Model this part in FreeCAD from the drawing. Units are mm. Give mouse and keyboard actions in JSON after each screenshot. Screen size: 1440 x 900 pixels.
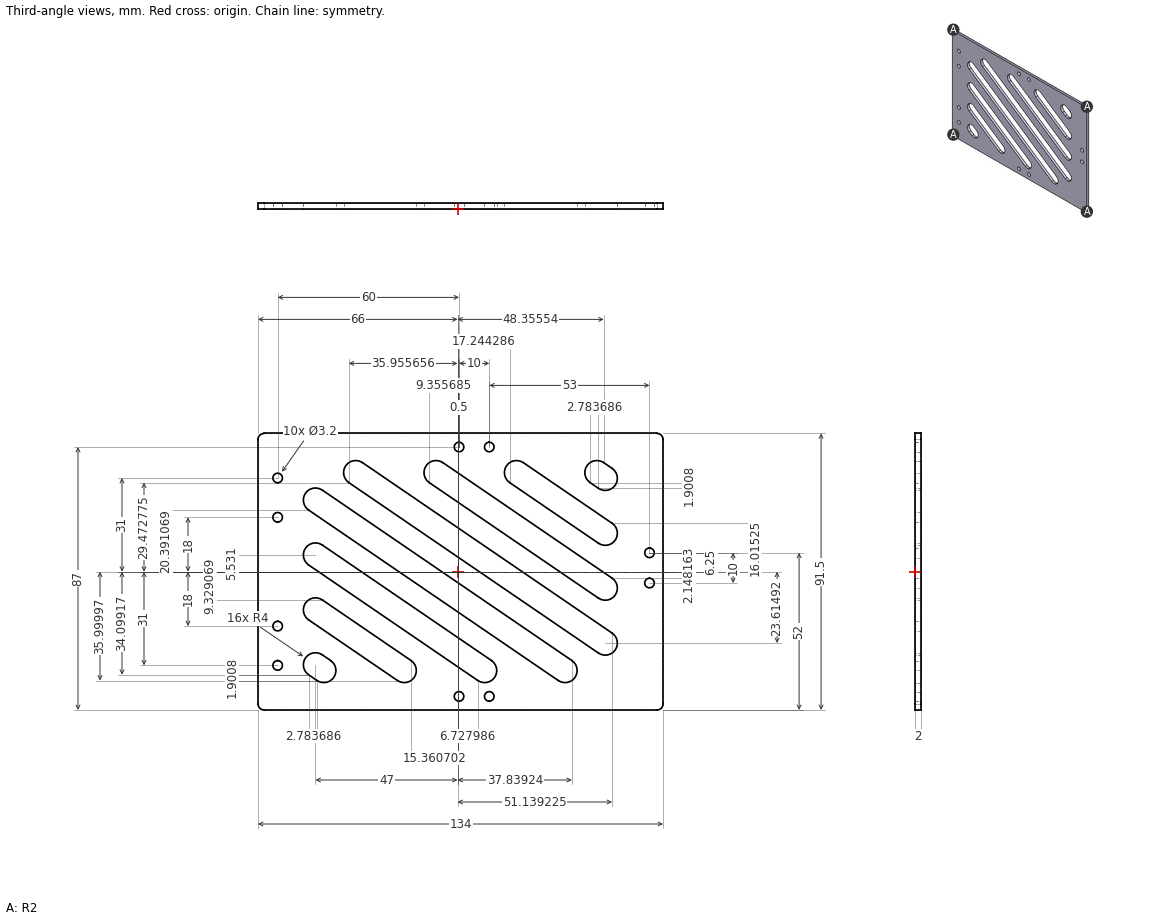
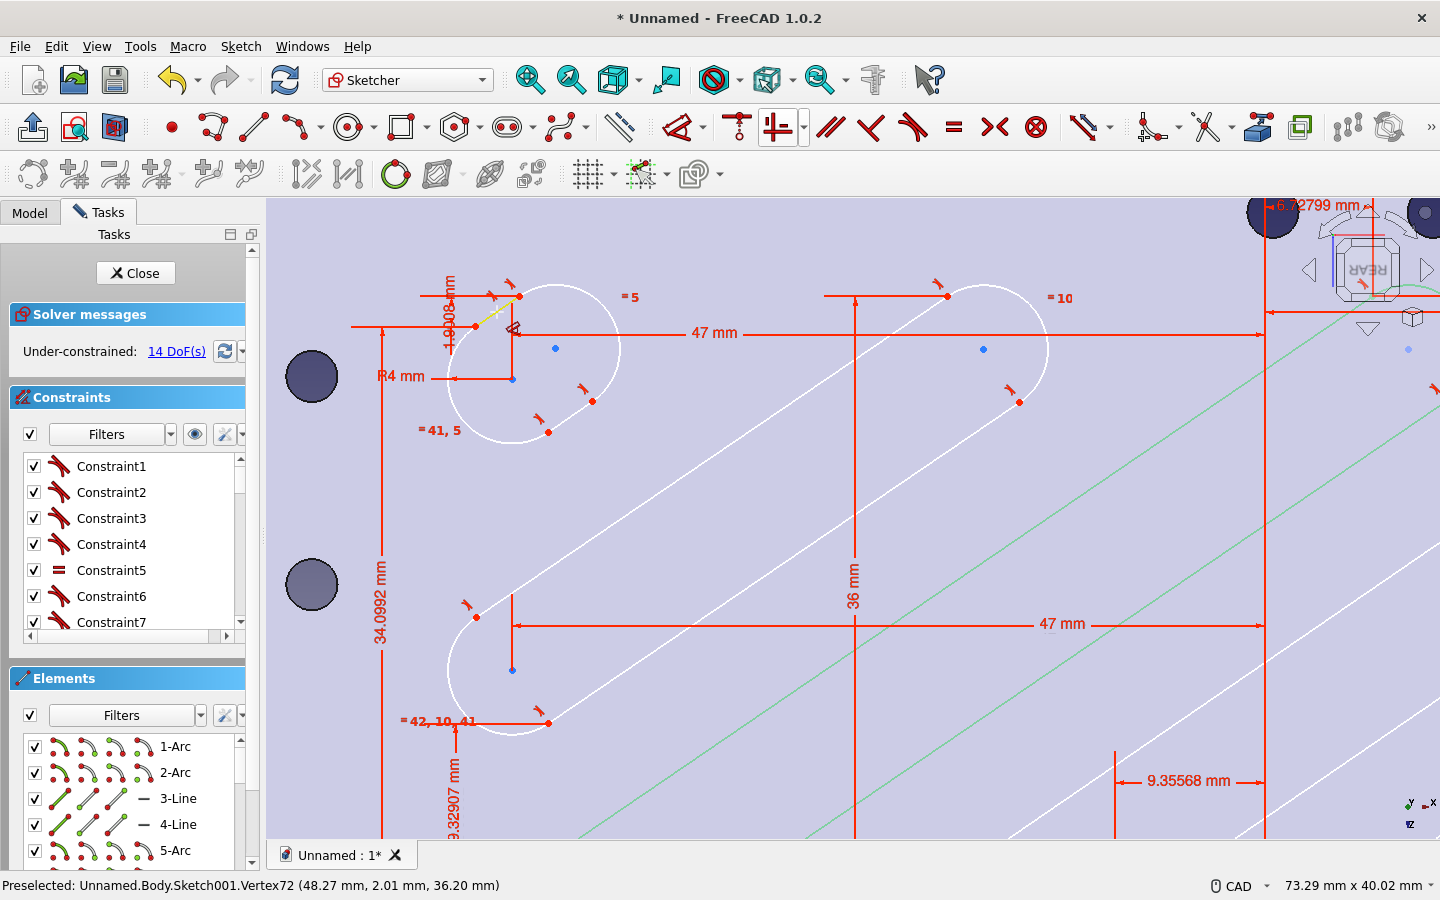
{"action": "left_click", "coordinate": [497, 312]}
{"action": "left_click", "coordinate": [497, 262]}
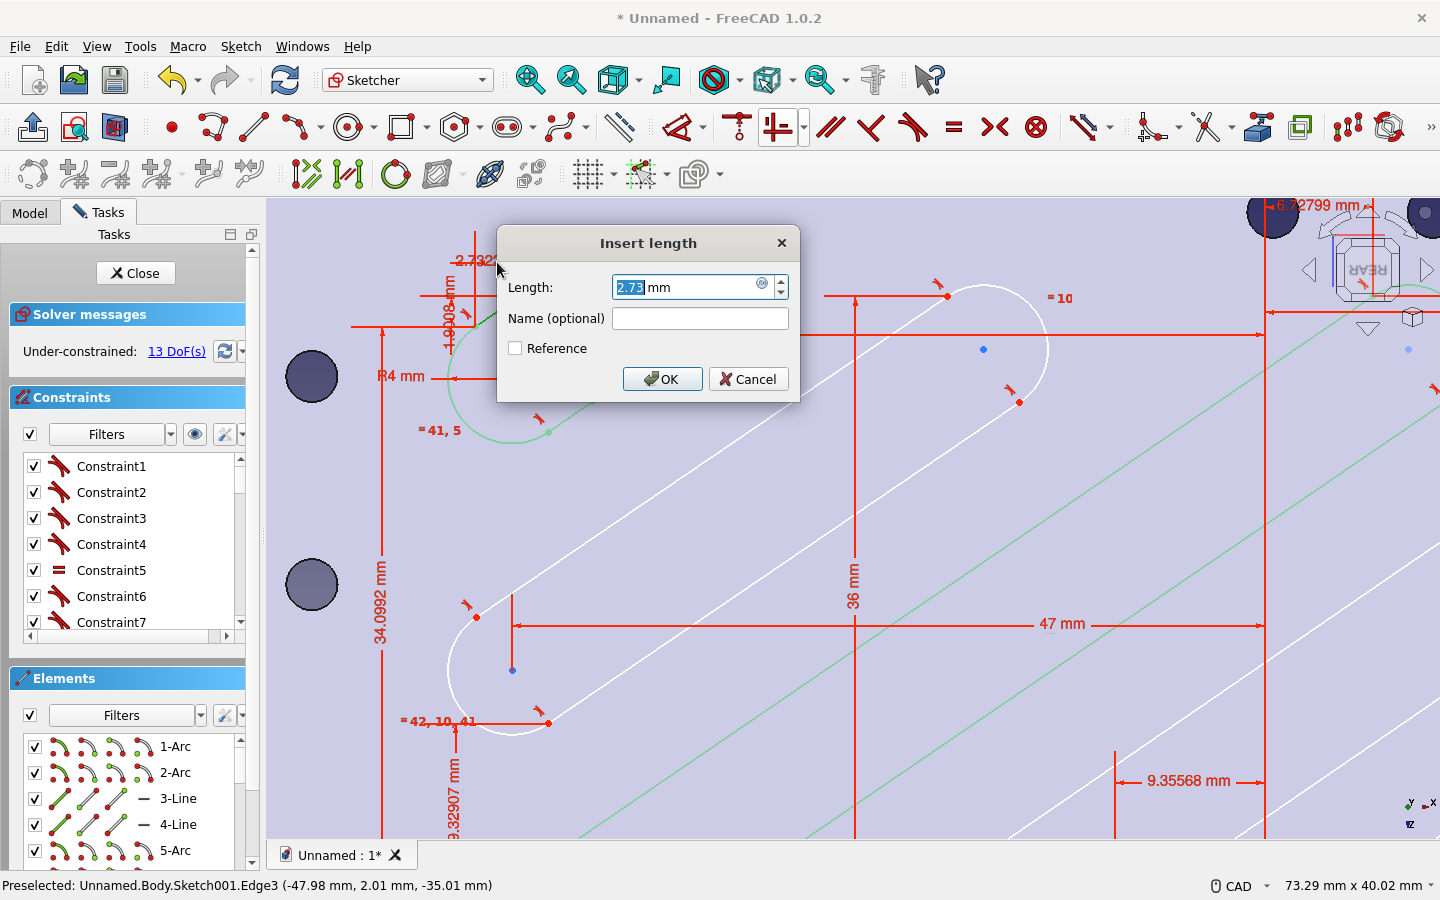
{"action": "type", "text": "2.783686"}
{"action": "key", "text": "Return"}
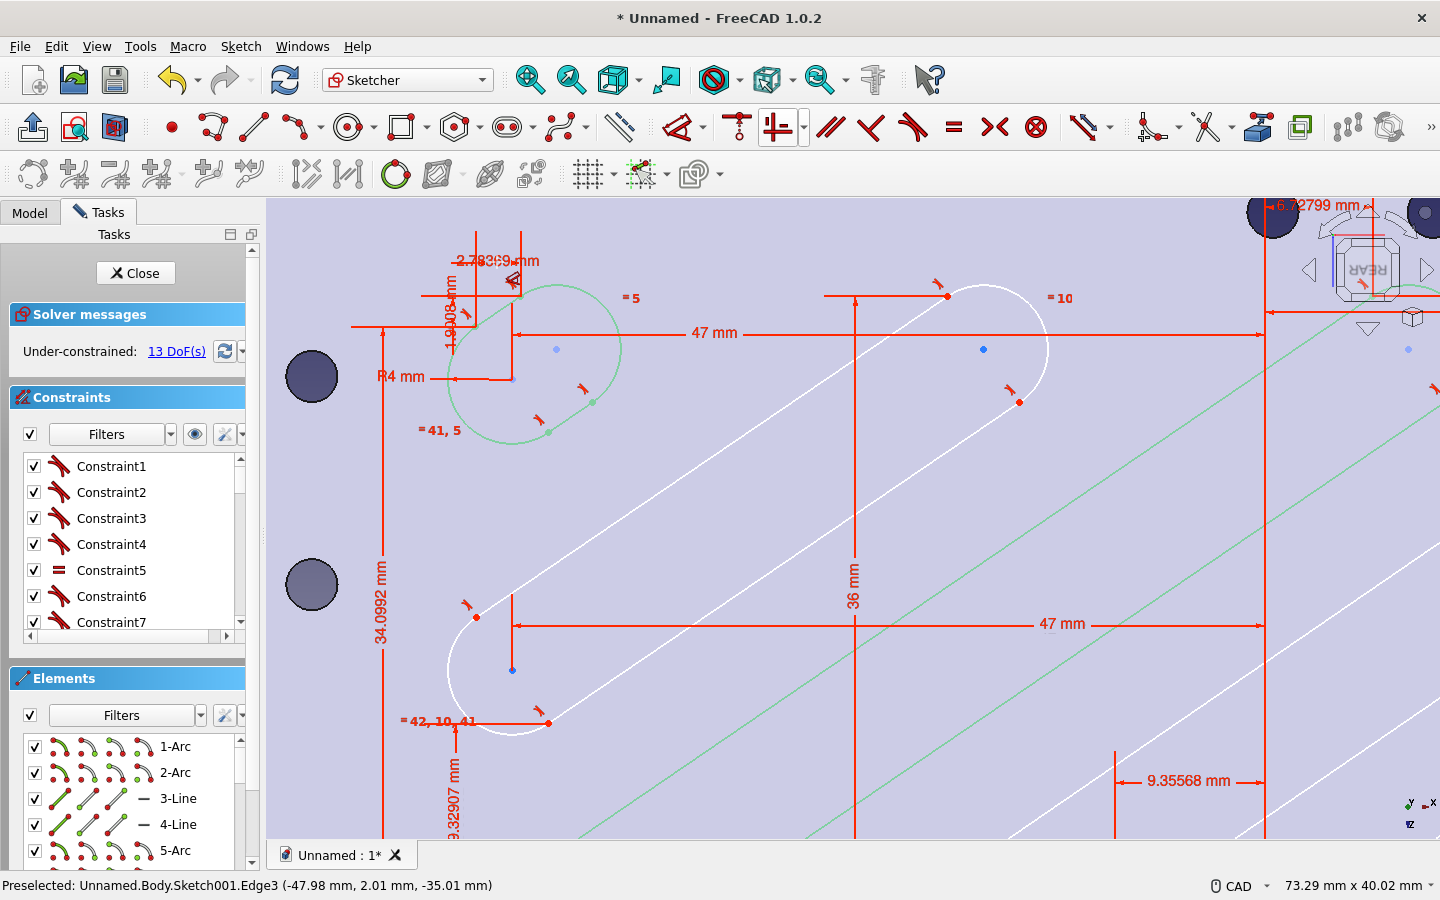
{"action": "scroll", "coordinate": [496, 312], "scroll_direction": "down", "scroll_amount": 5}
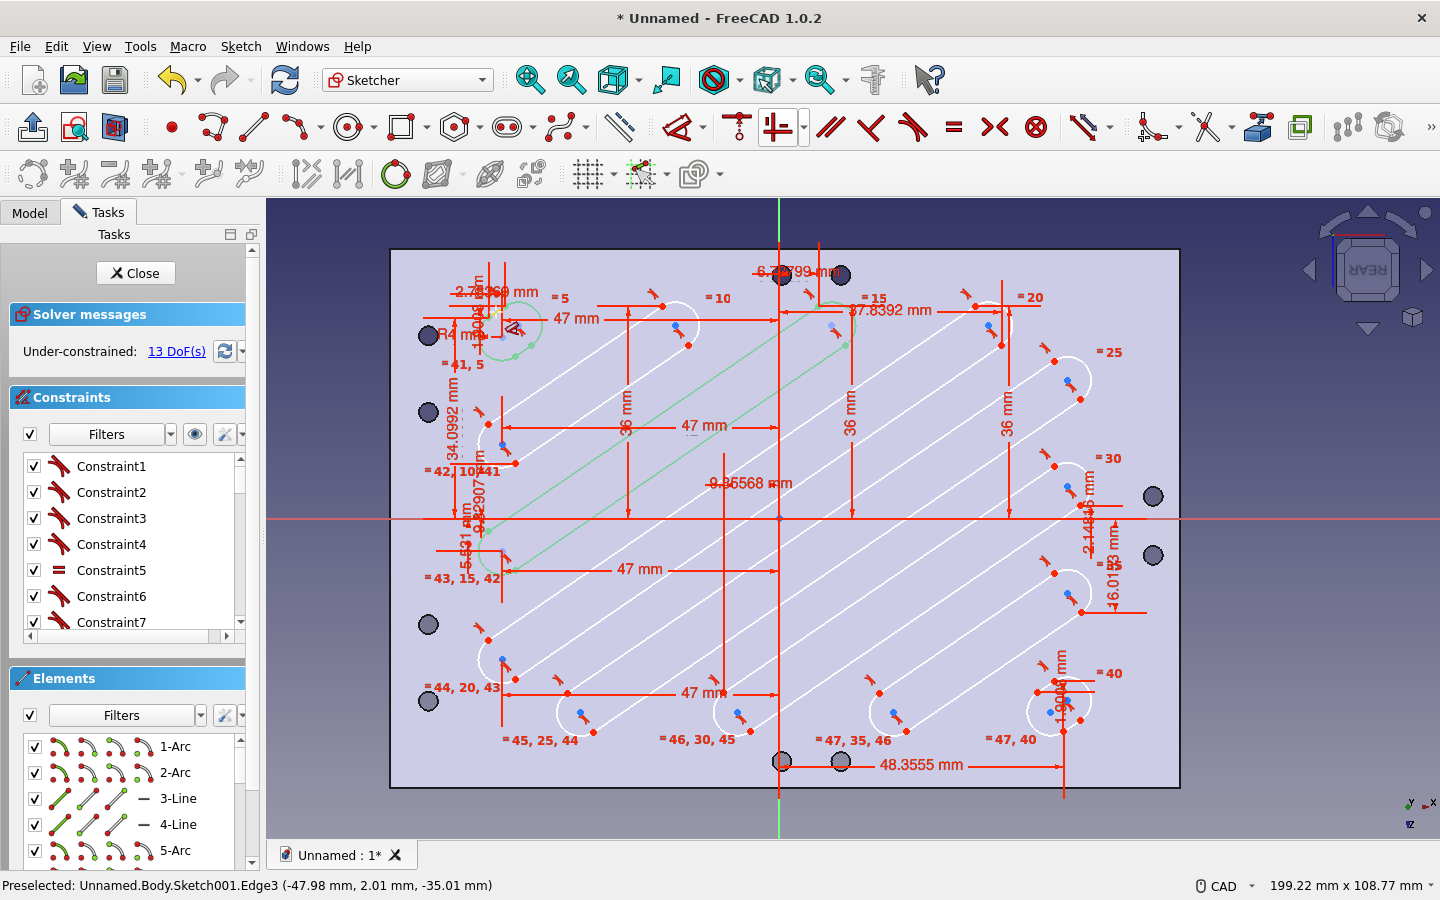
{"action": "scroll", "coordinate": [1043, 689], "scroll_direction": "up", "scroll_amount": 5}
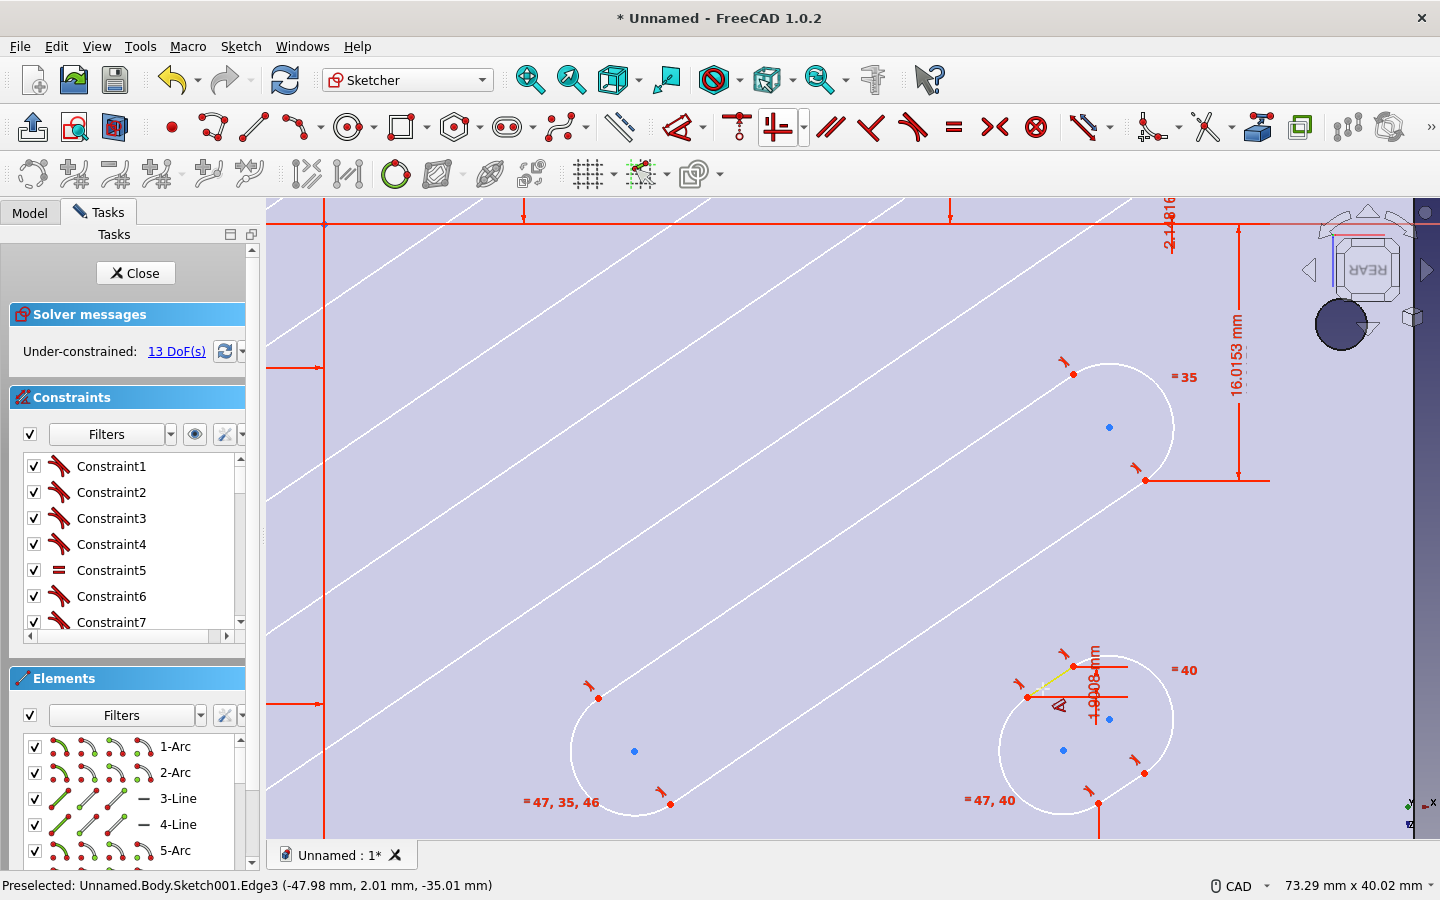
{"action": "left_click", "coordinate": [1042, 688]}
{"action": "left_click", "coordinate": [1051, 731]}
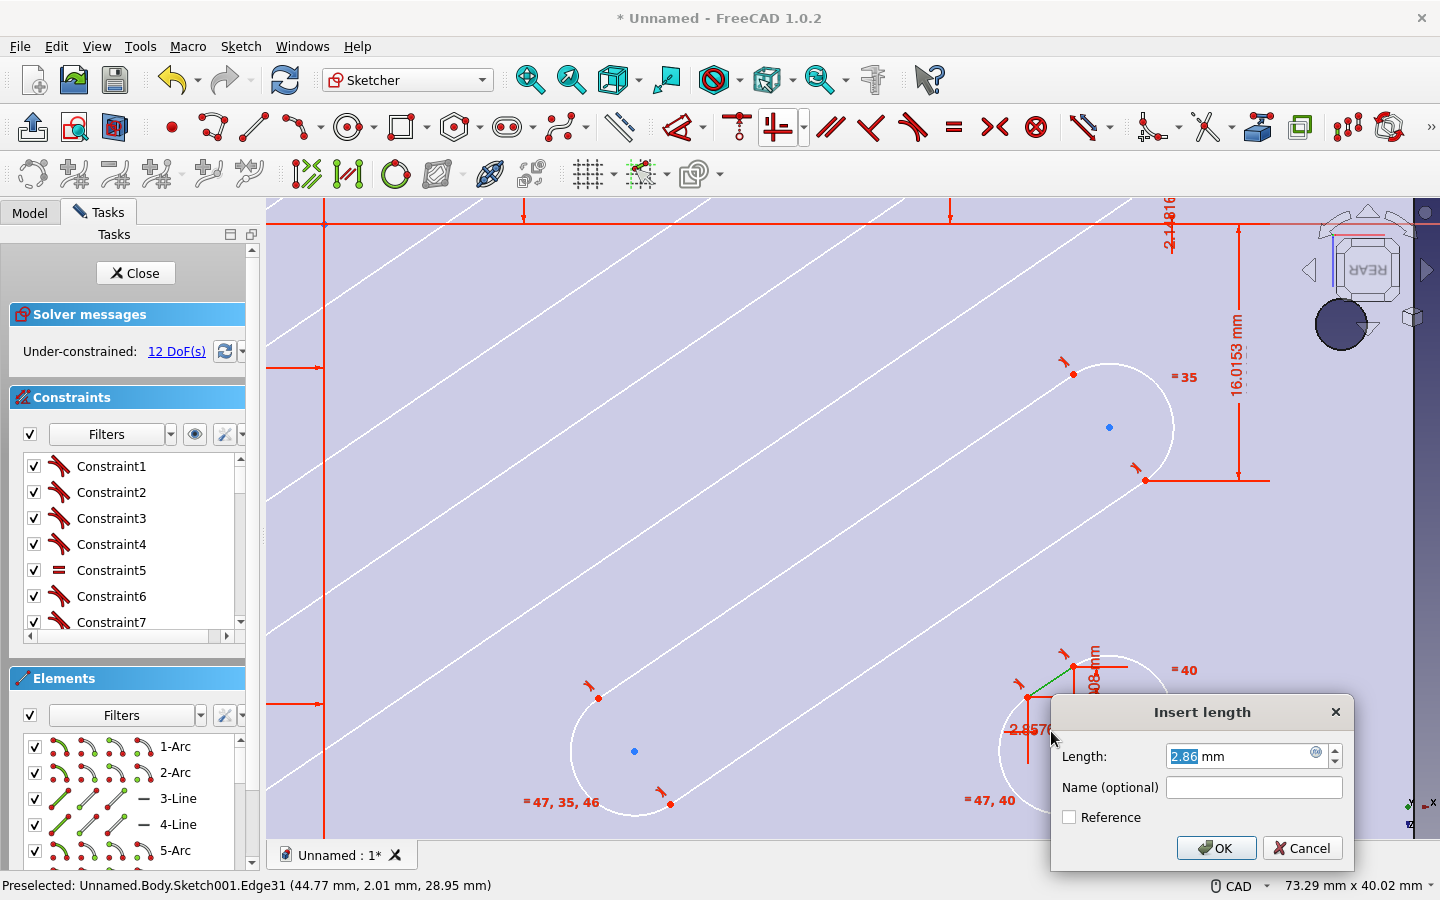
{"action": "type", "text": "2.783686"}
{"action": "key", "text": "Return"}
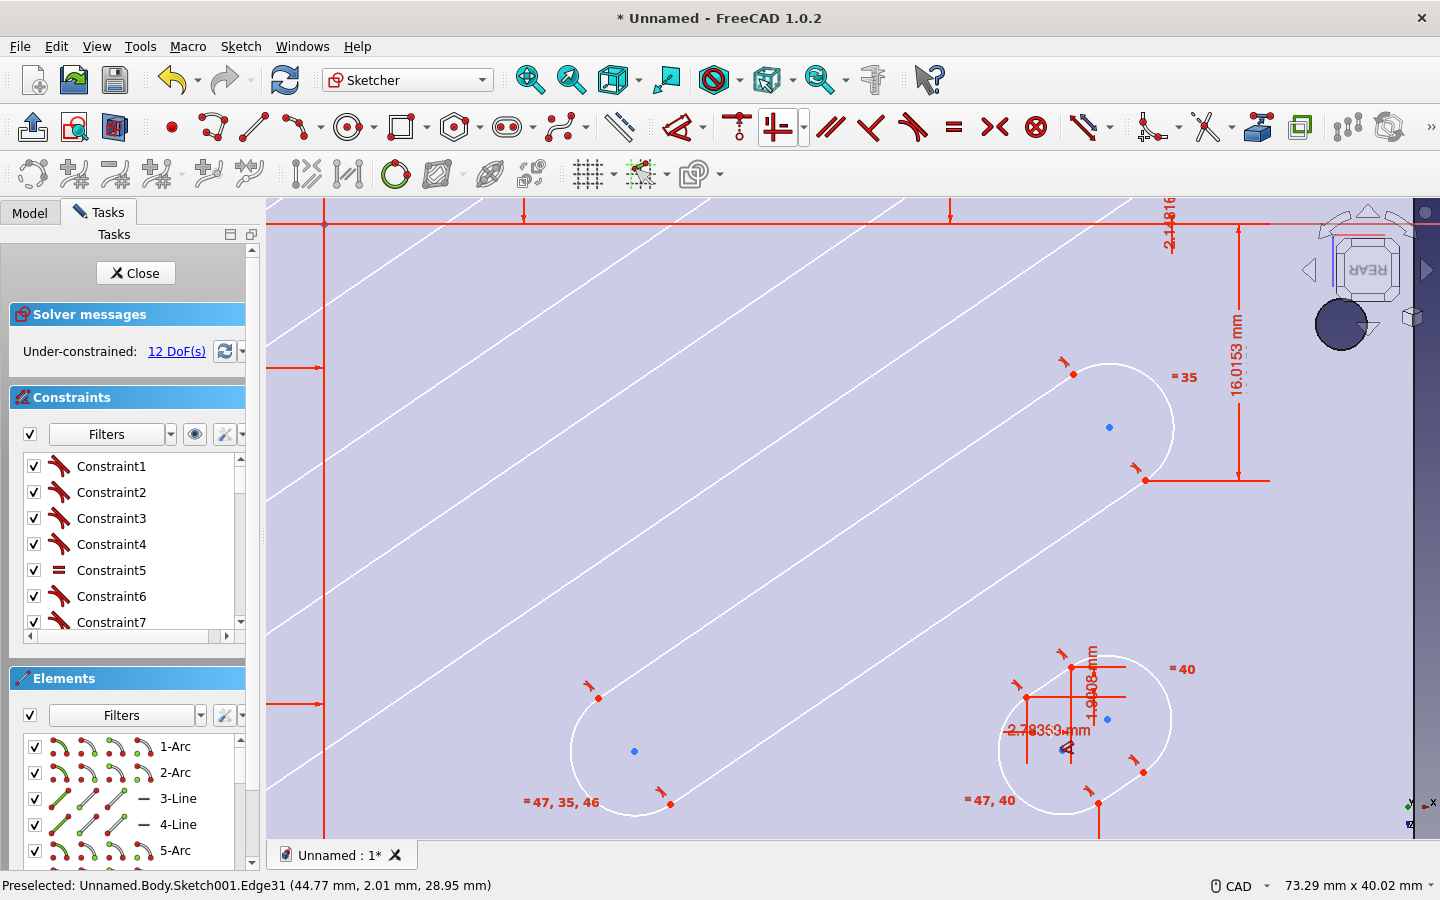
{"action": "scroll", "coordinate": [1044, 689], "scroll_direction": "down", "scroll_amount": 5}